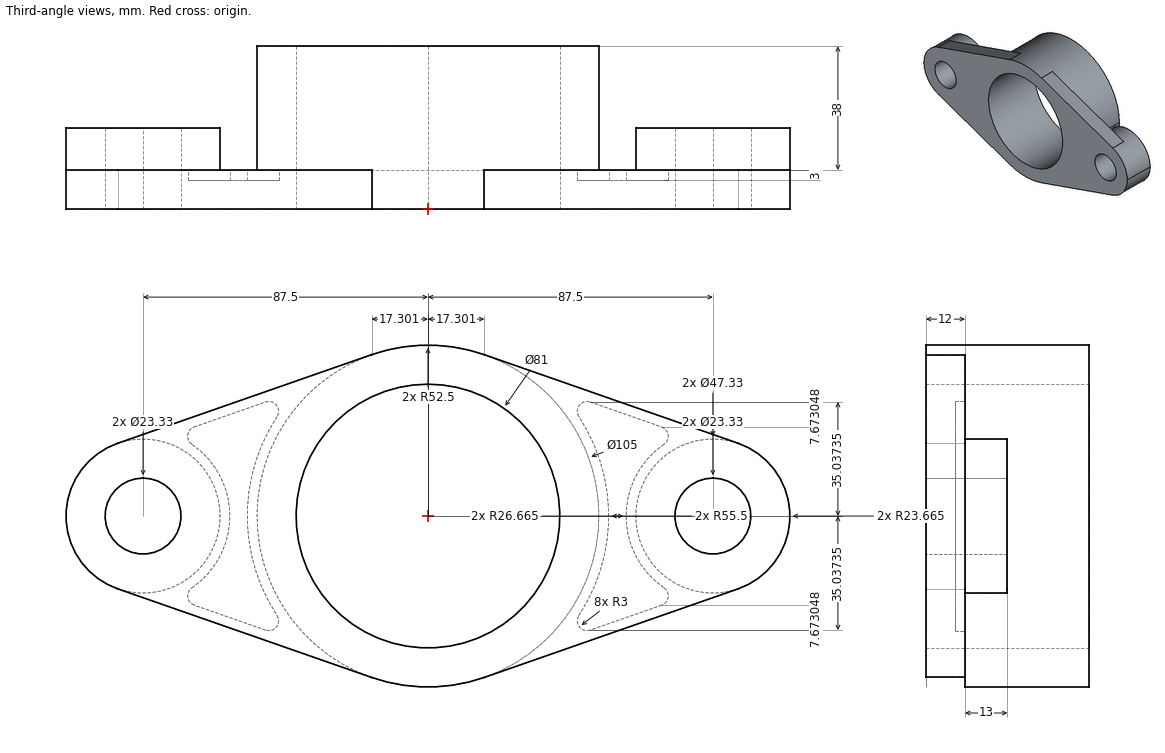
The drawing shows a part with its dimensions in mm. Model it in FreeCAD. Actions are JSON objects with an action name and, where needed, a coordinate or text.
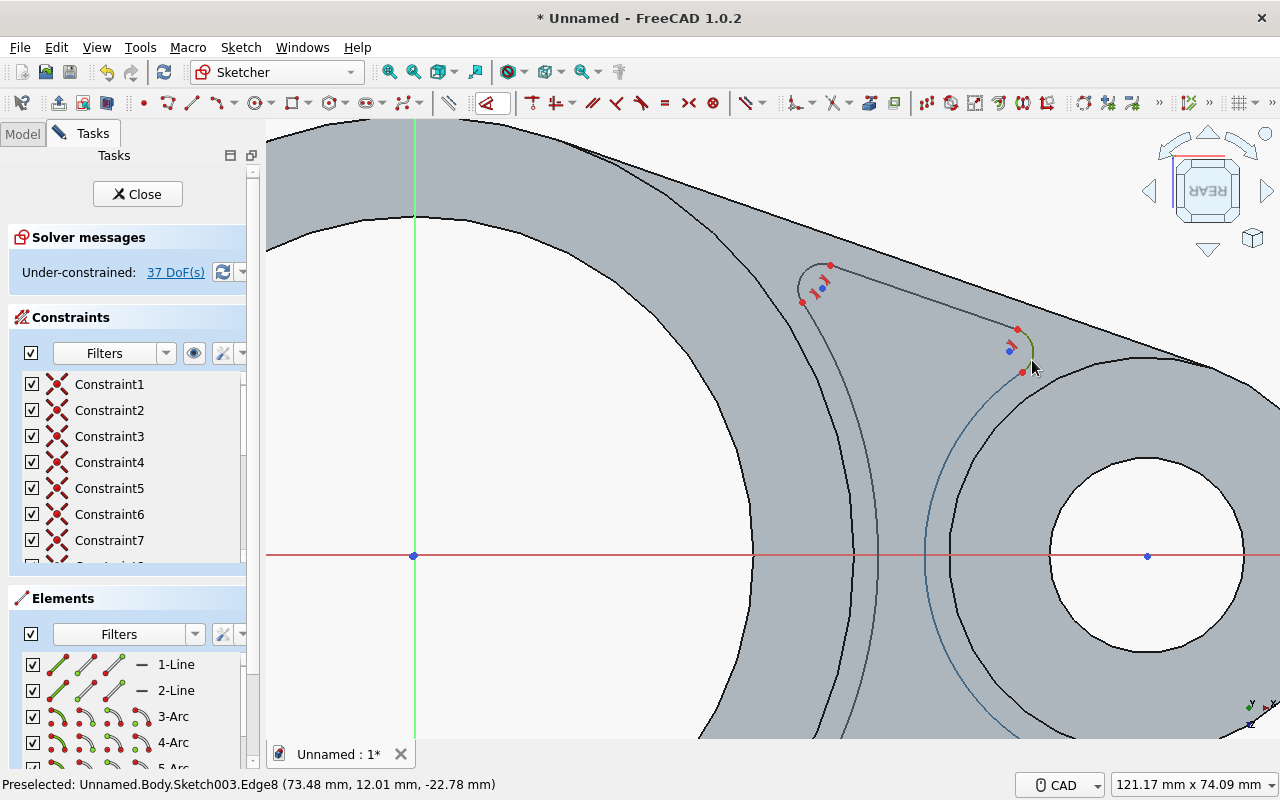
{"action": "left_click", "coordinate": [642, 104]}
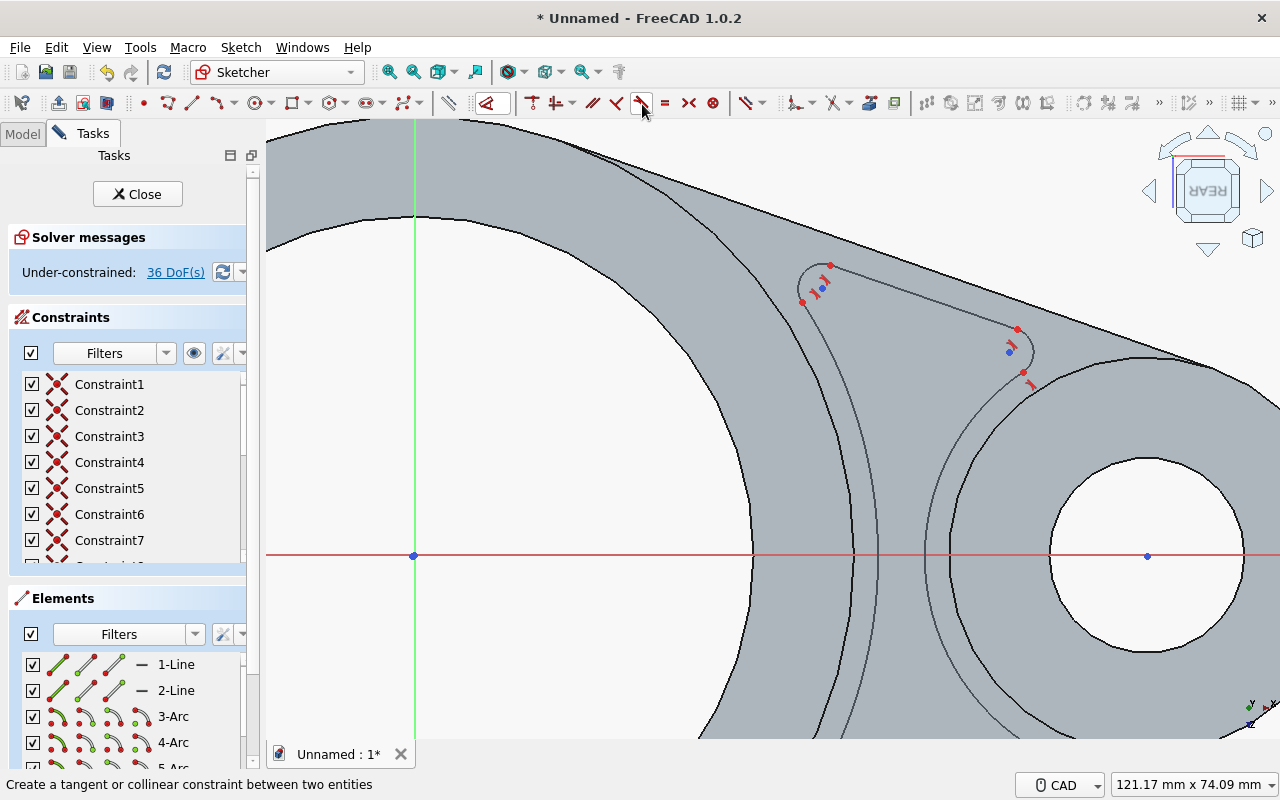
{"action": "scroll", "coordinate": [941, 326], "scroll_direction": "down", "scroll_amount": 4}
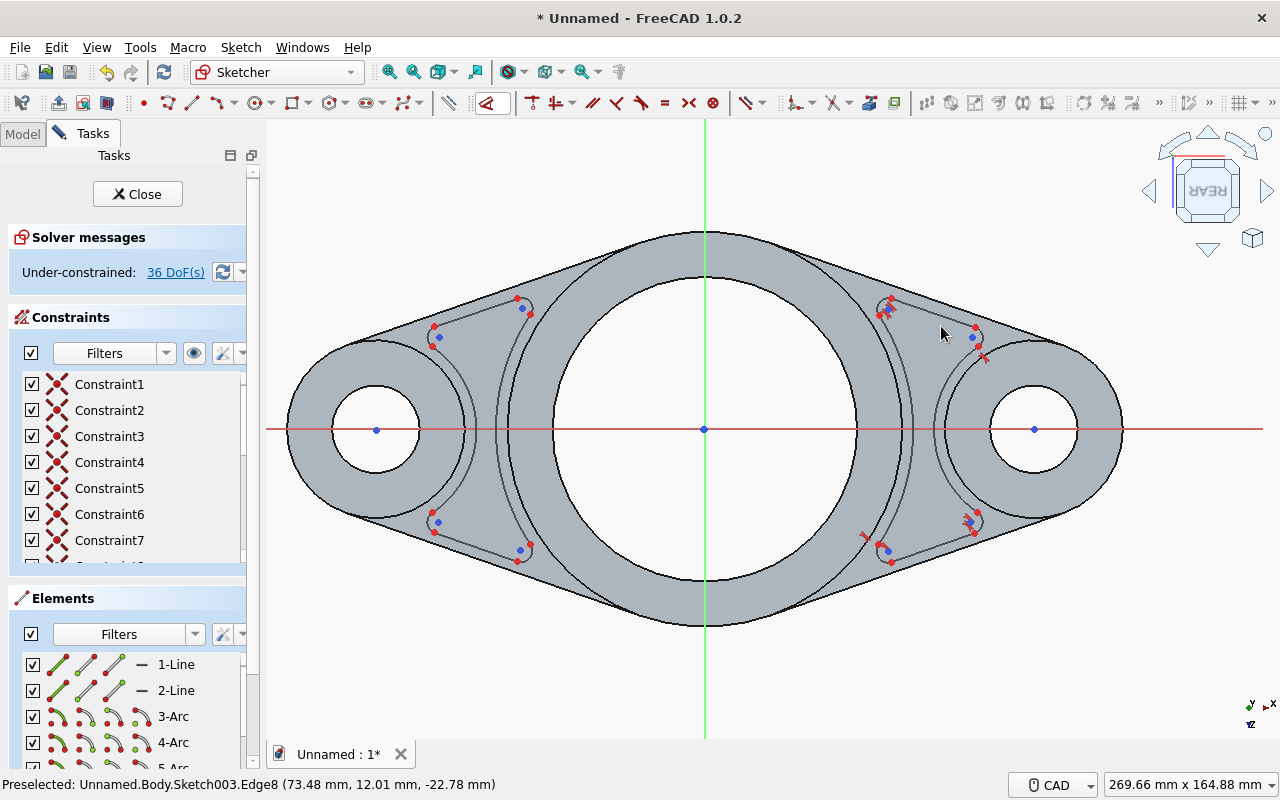
{"action": "left_click", "coordinate": [460, 542]}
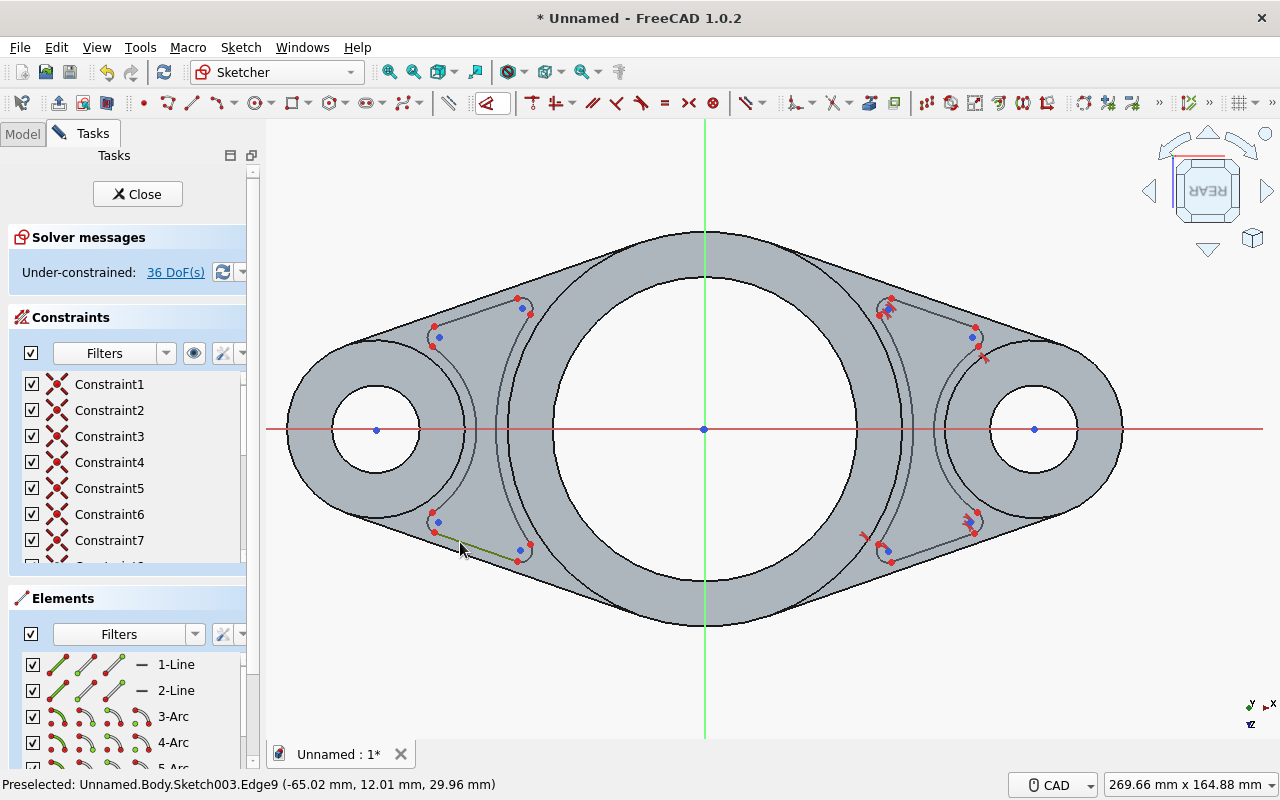
{"action": "left_click", "coordinate": [530, 558]}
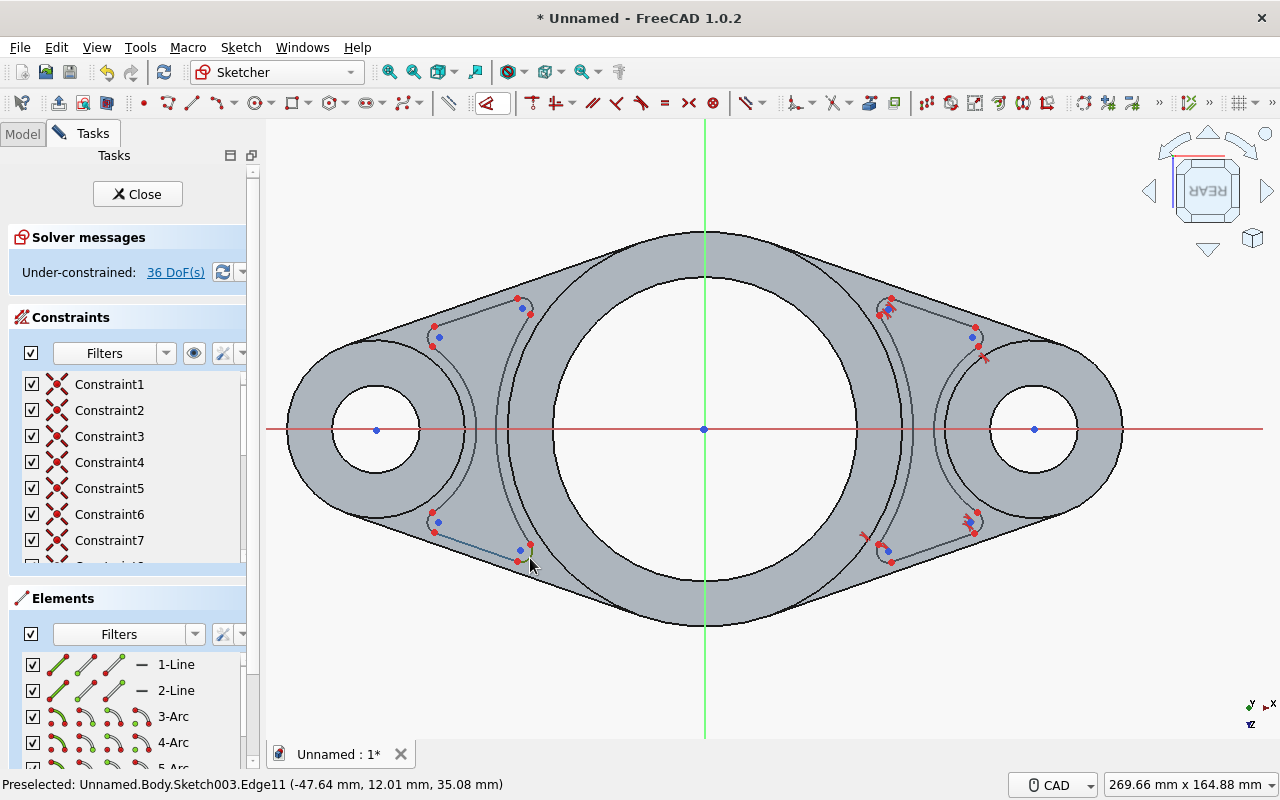
{"action": "left_click", "coordinate": [642, 104]}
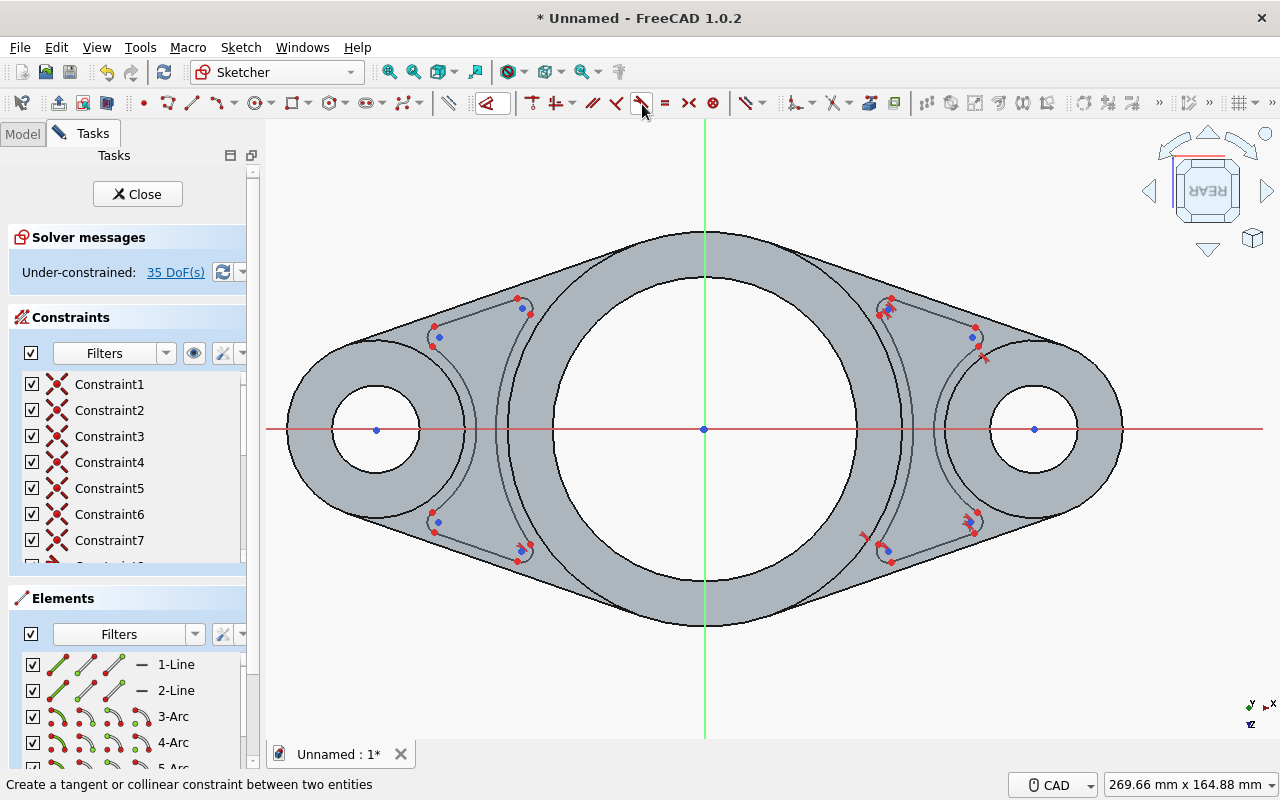
{"action": "left_click", "coordinate": [460, 542]}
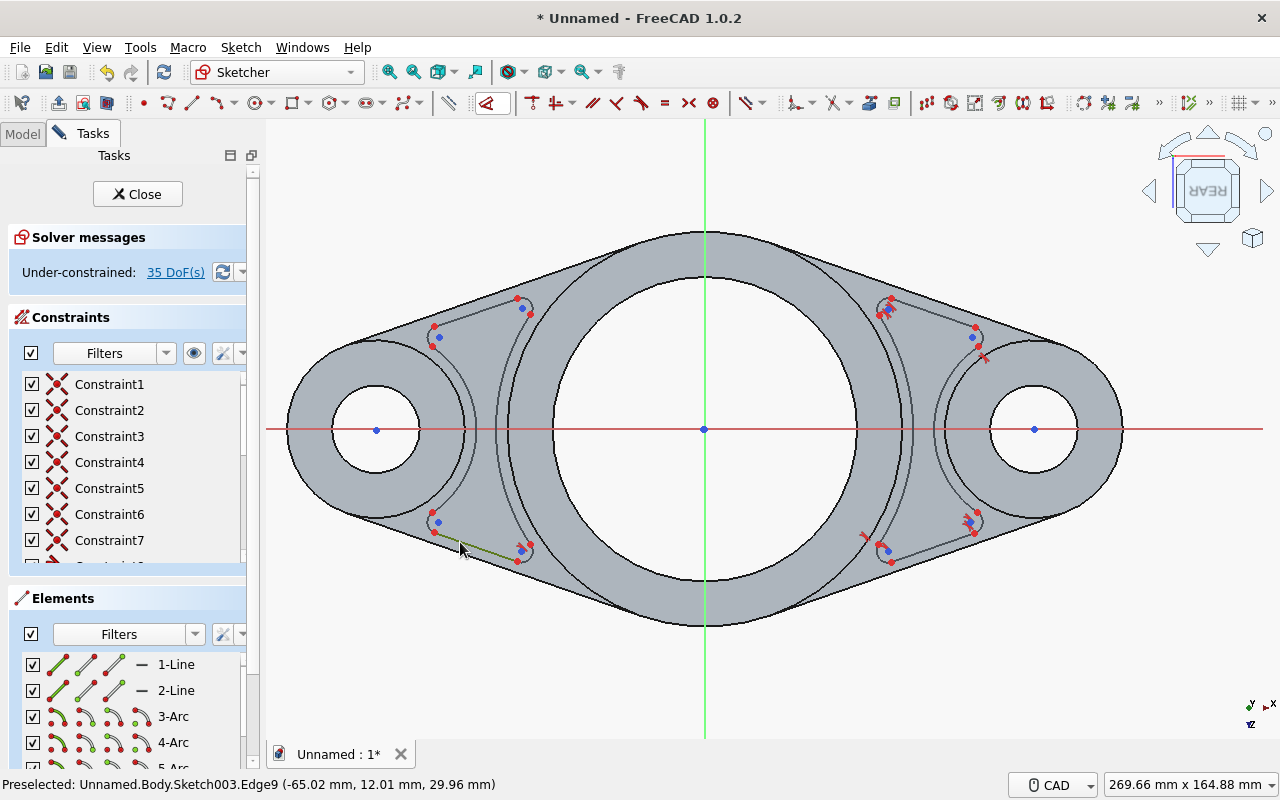
{"action": "left_click", "coordinate": [427, 524]}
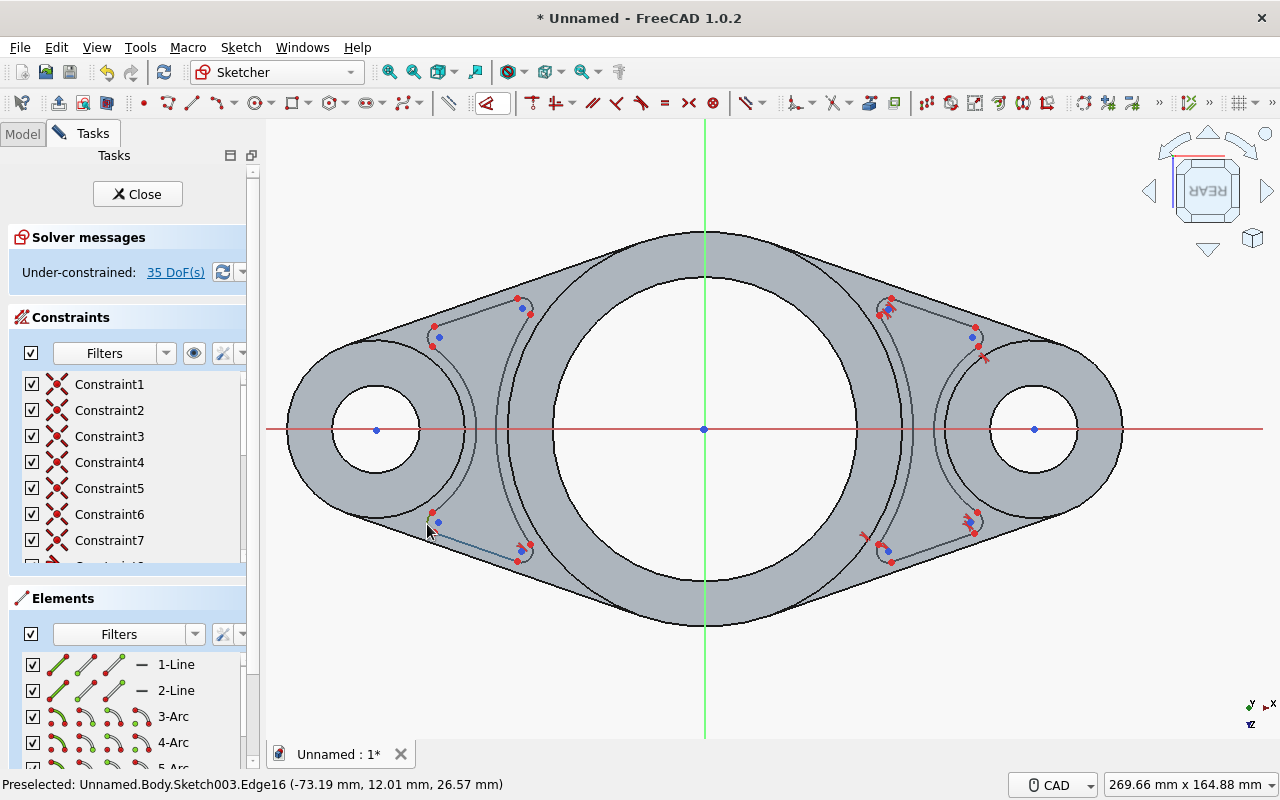
{"action": "left_click", "coordinate": [642, 104]}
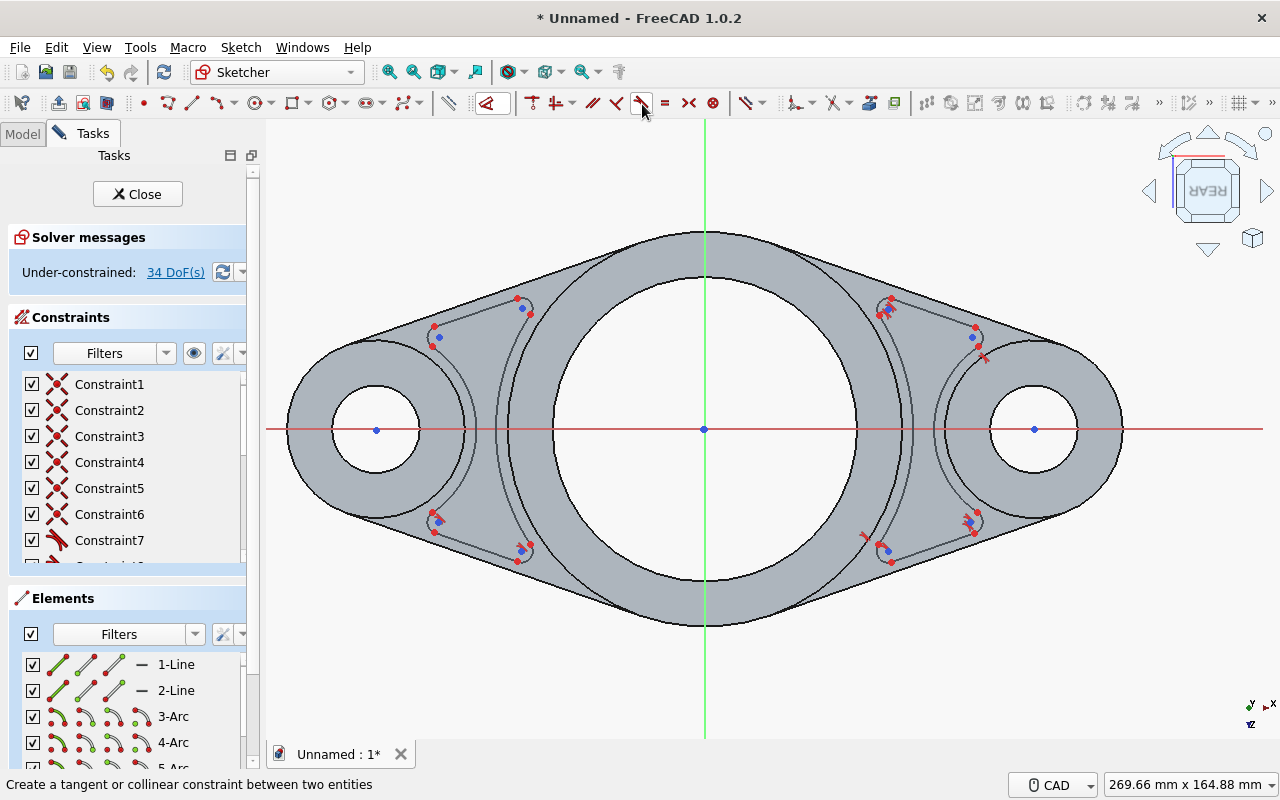
{"action": "left_click", "coordinate": [493, 307]}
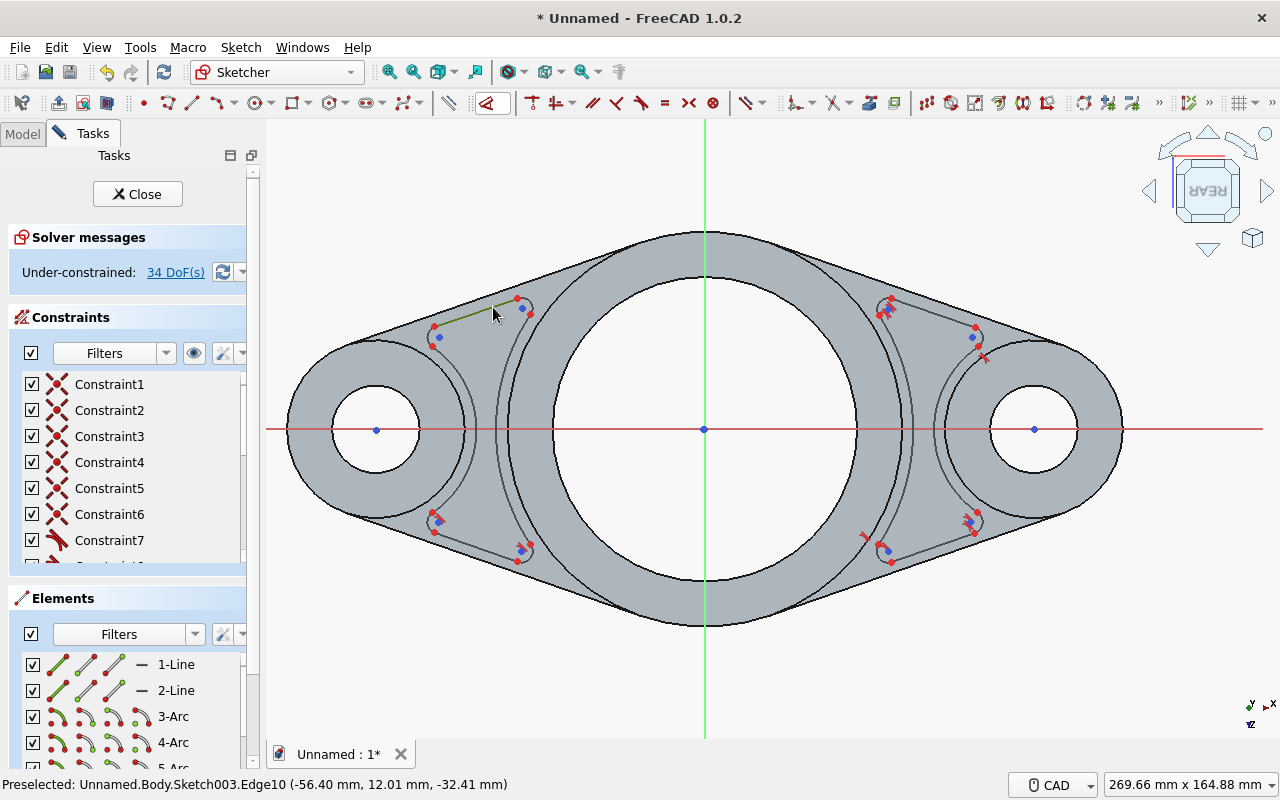
{"action": "scroll", "coordinate": [530, 302], "scroll_direction": "up", "scroll_amount": 2}